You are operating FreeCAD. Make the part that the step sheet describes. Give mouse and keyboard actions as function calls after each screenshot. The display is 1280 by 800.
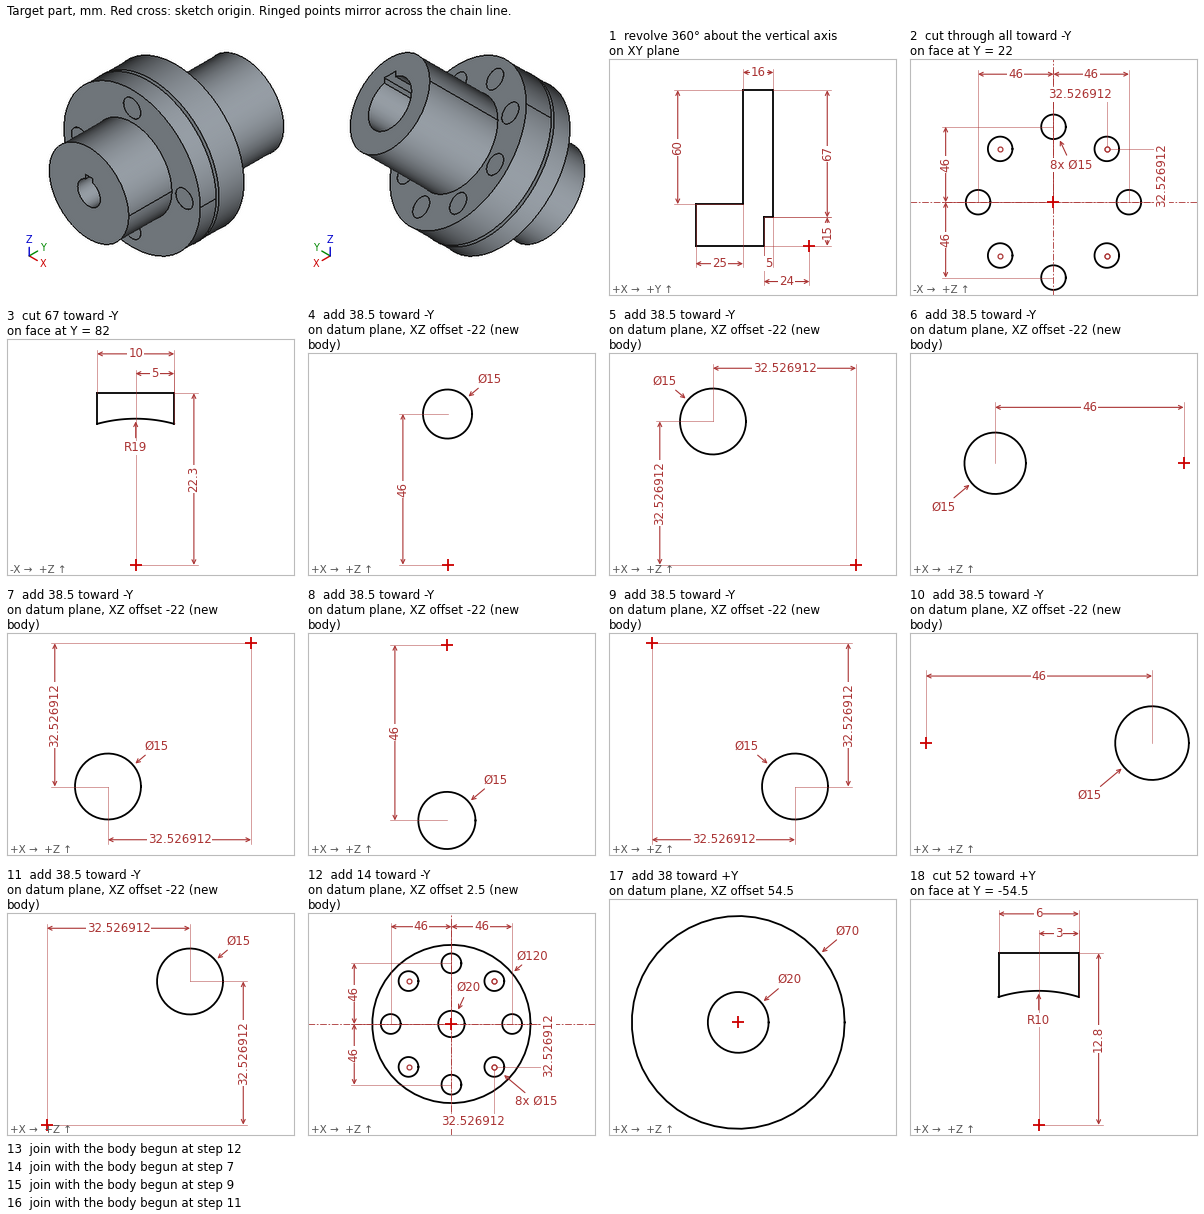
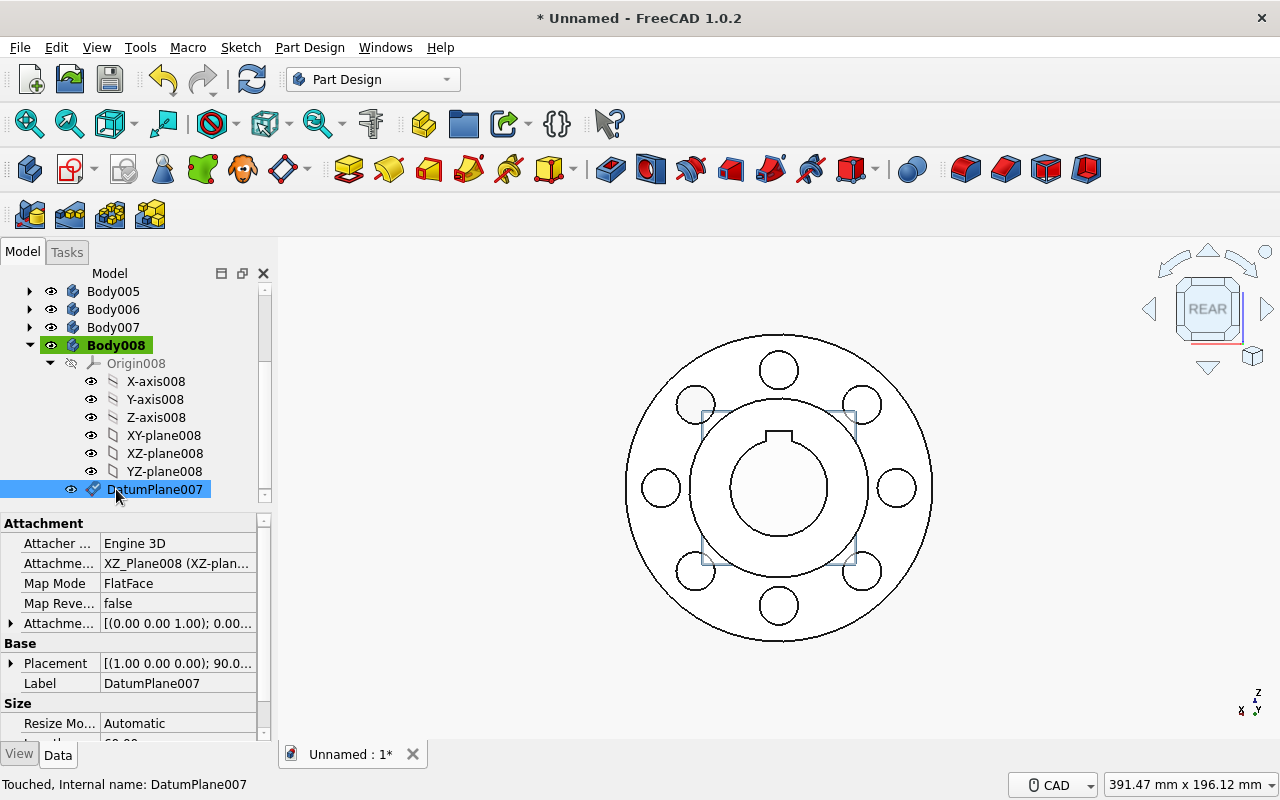
click(70, 170)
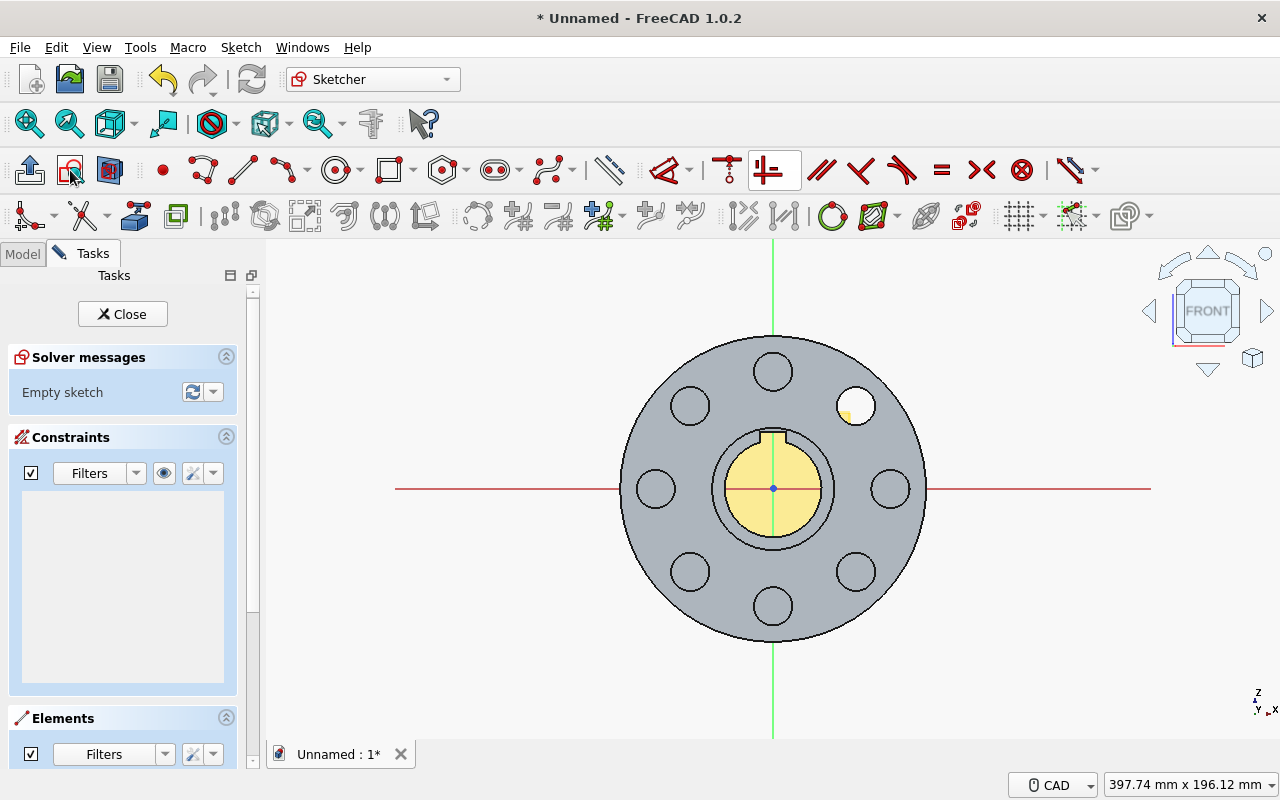
scroll(875, 396, up, 11)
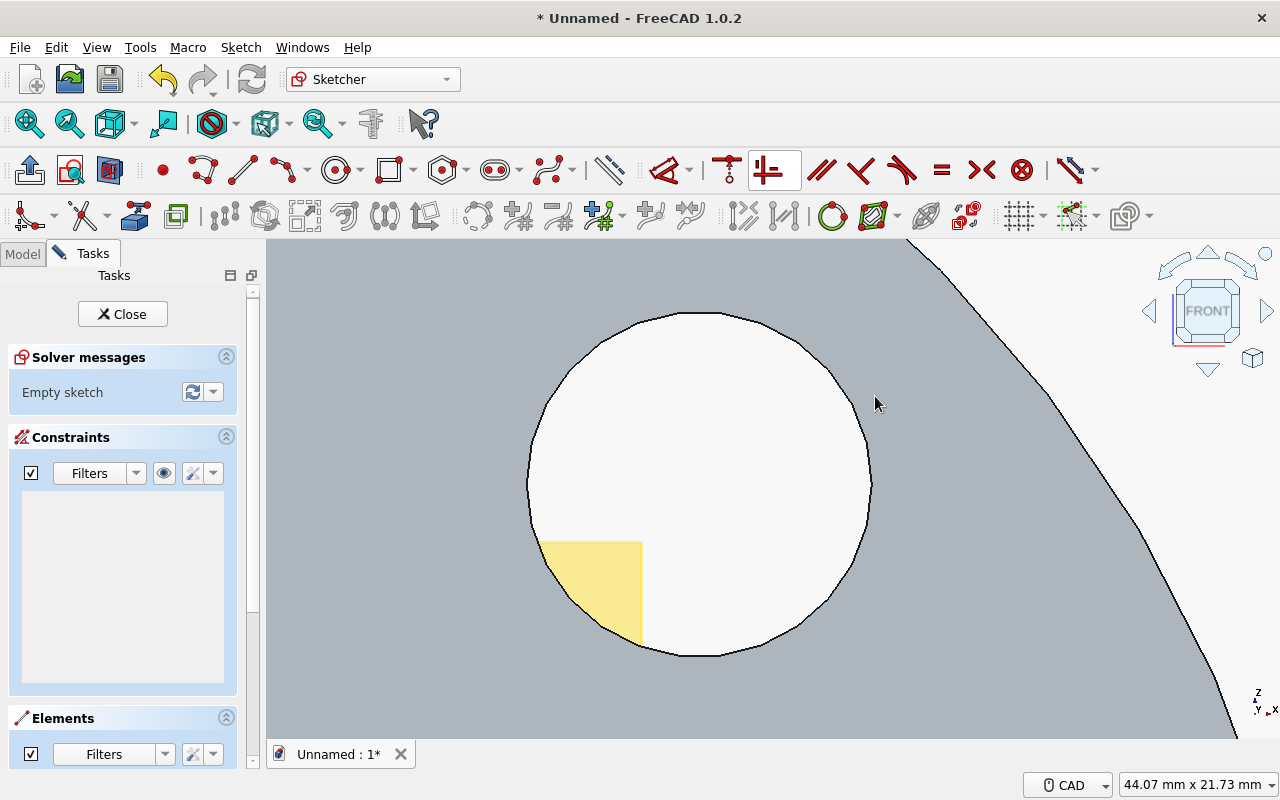
click(336, 170)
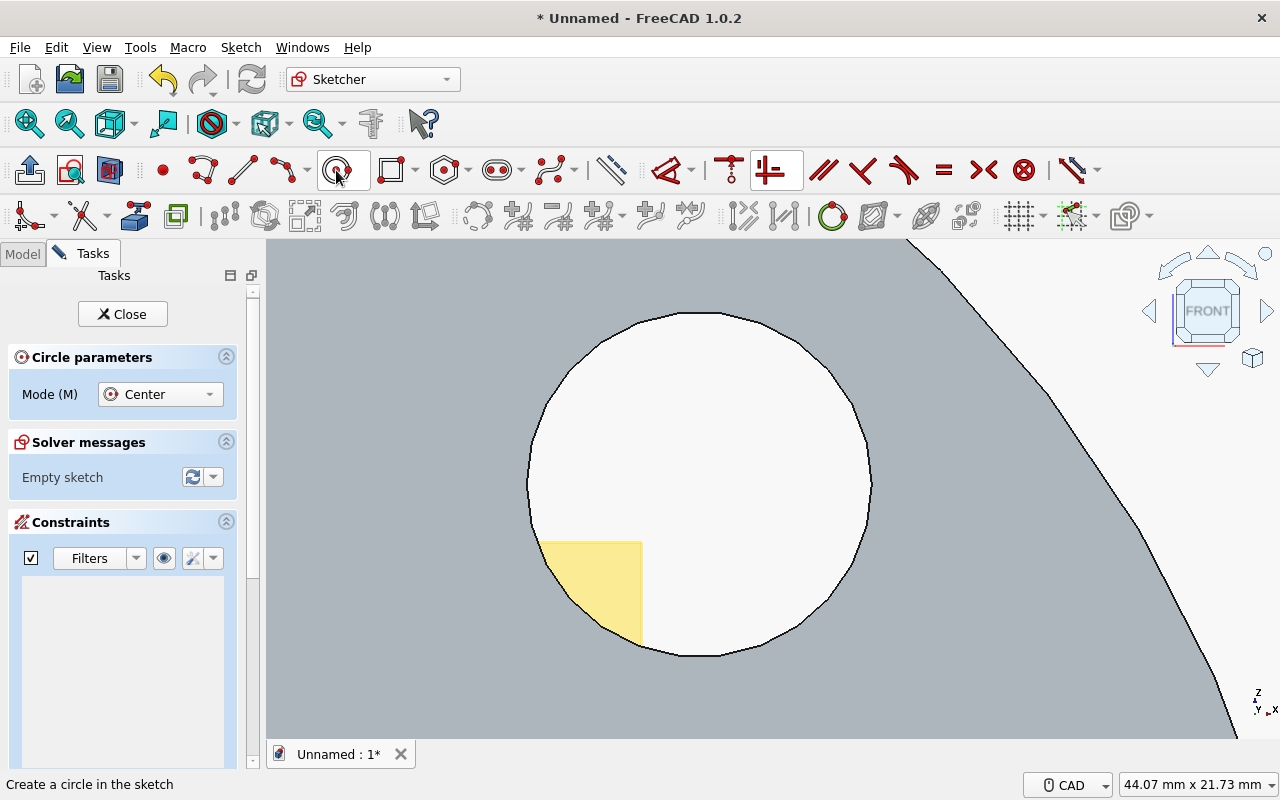
click(699, 484)
click(821, 362)
key(Escape)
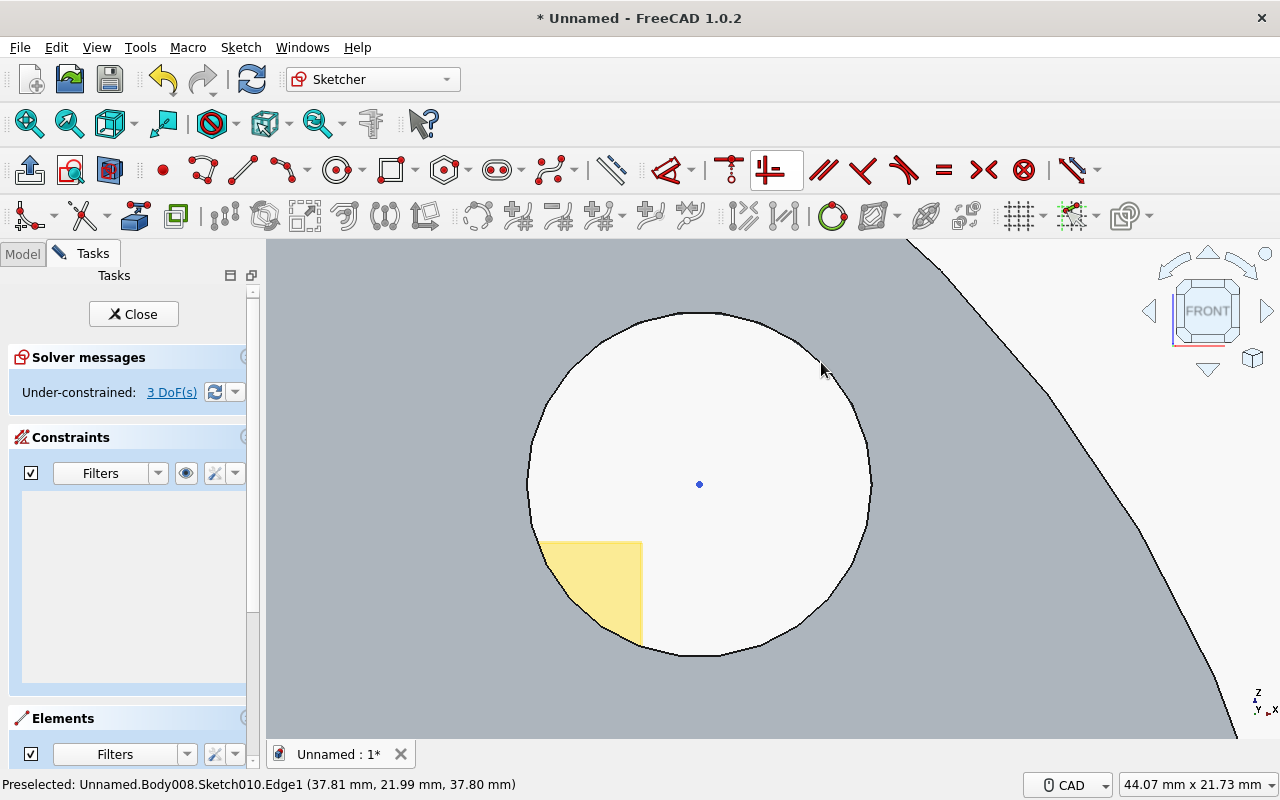
click(666, 170)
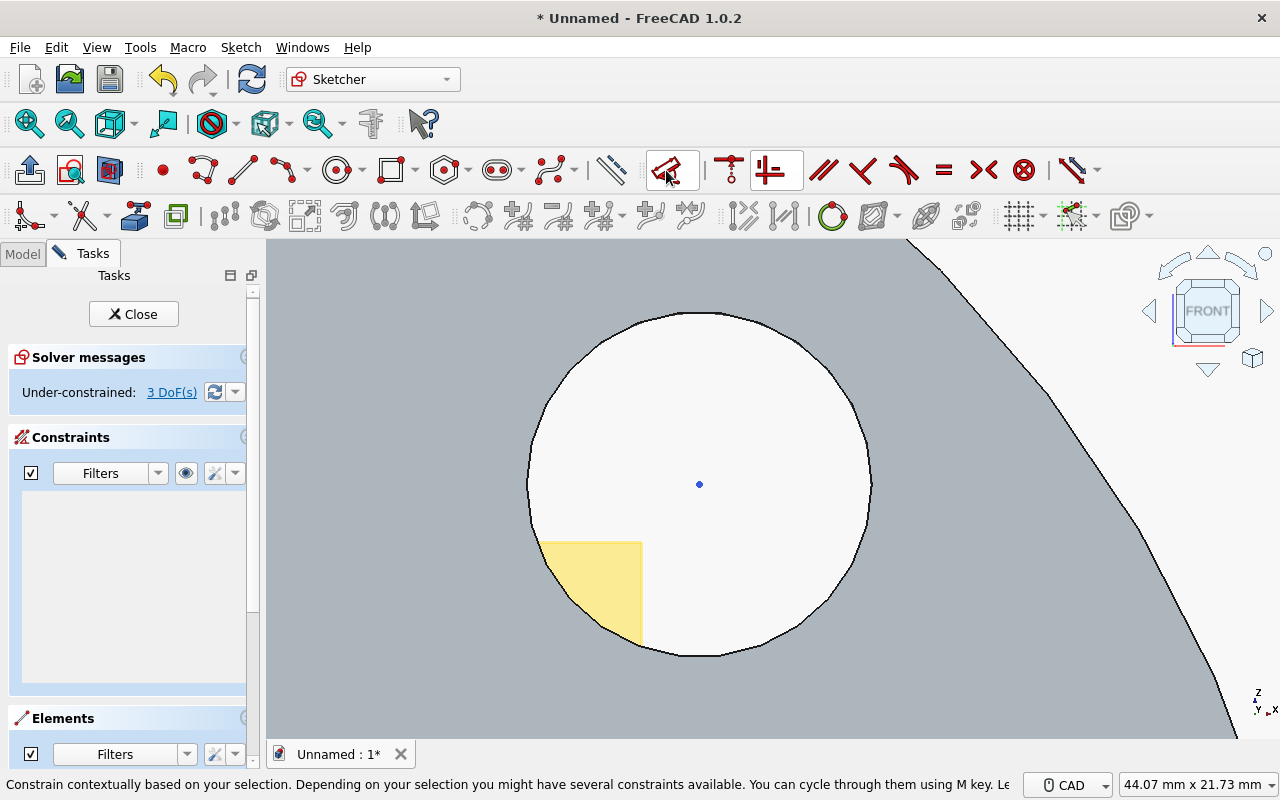
click(821, 363)
click(844, 340)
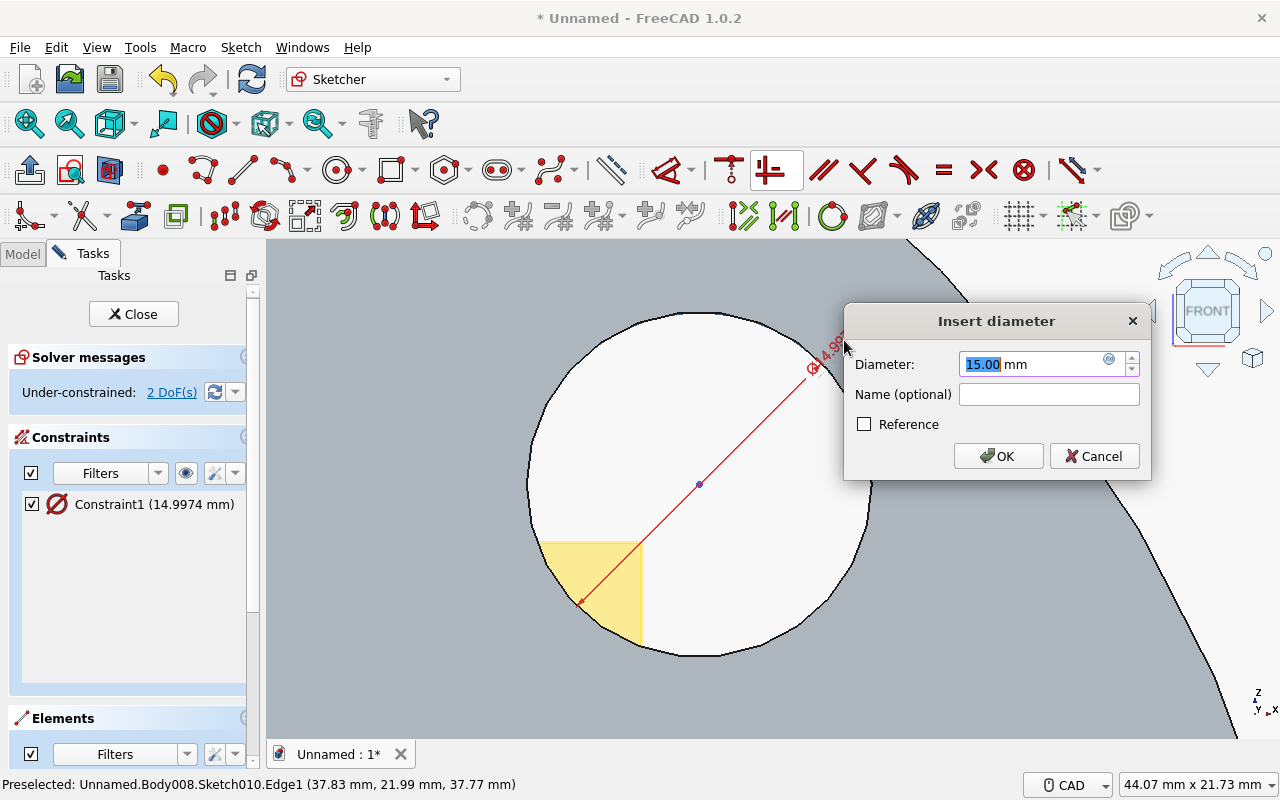
text(15)
key(Return)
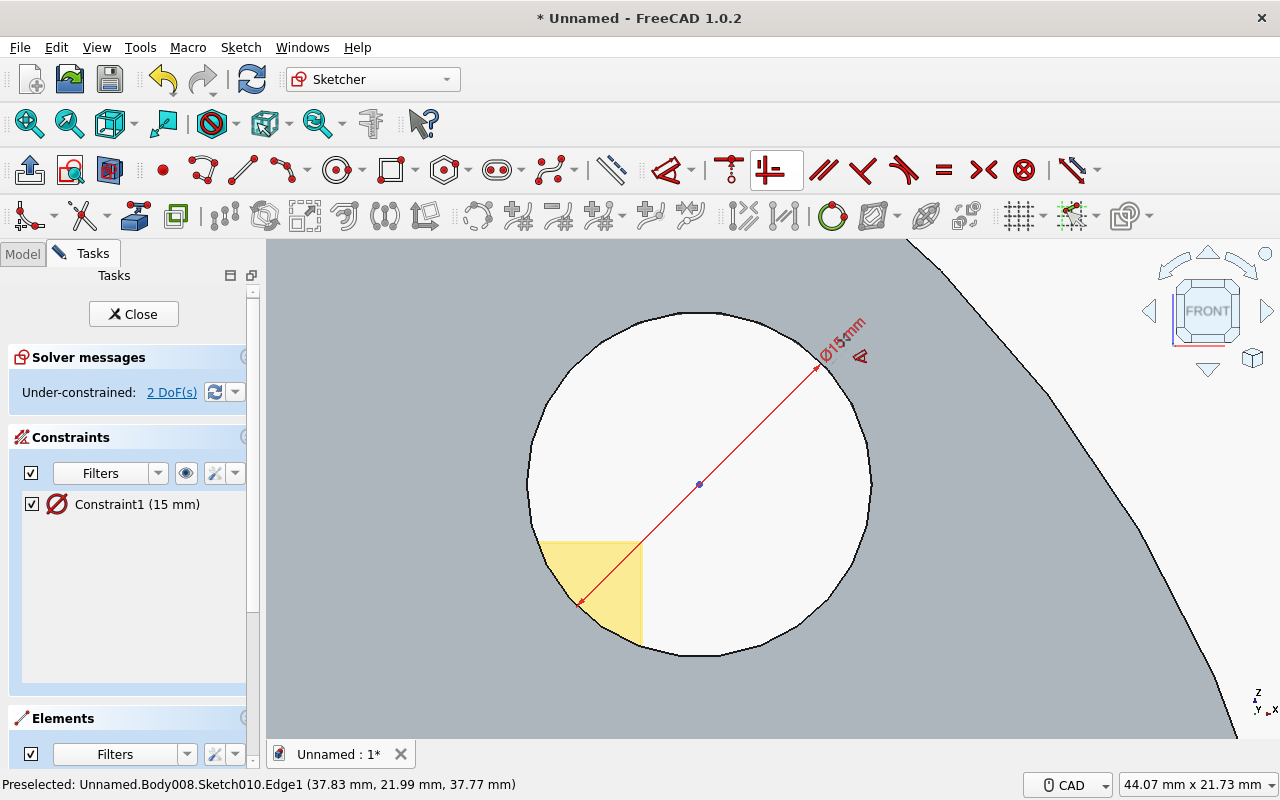
click(699, 485)
click(496, 451)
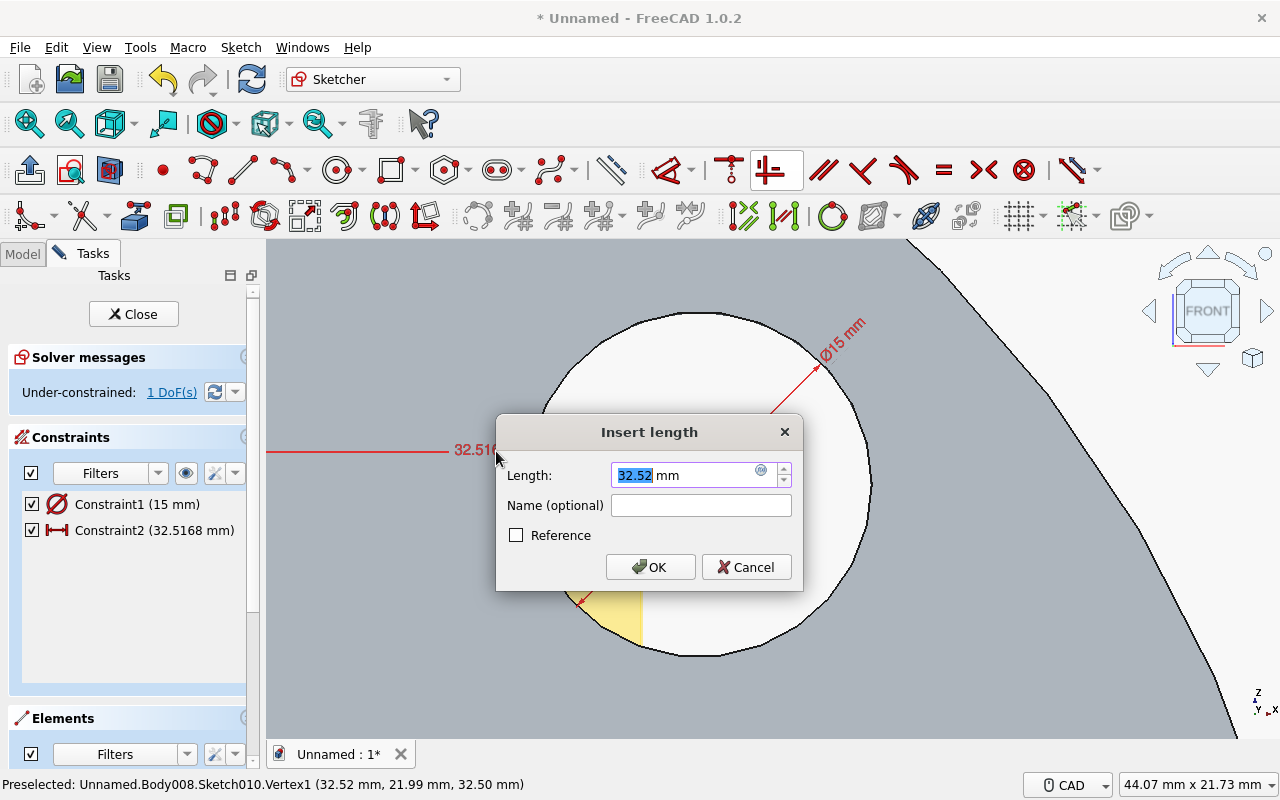
text(32.526912)
key(Return)